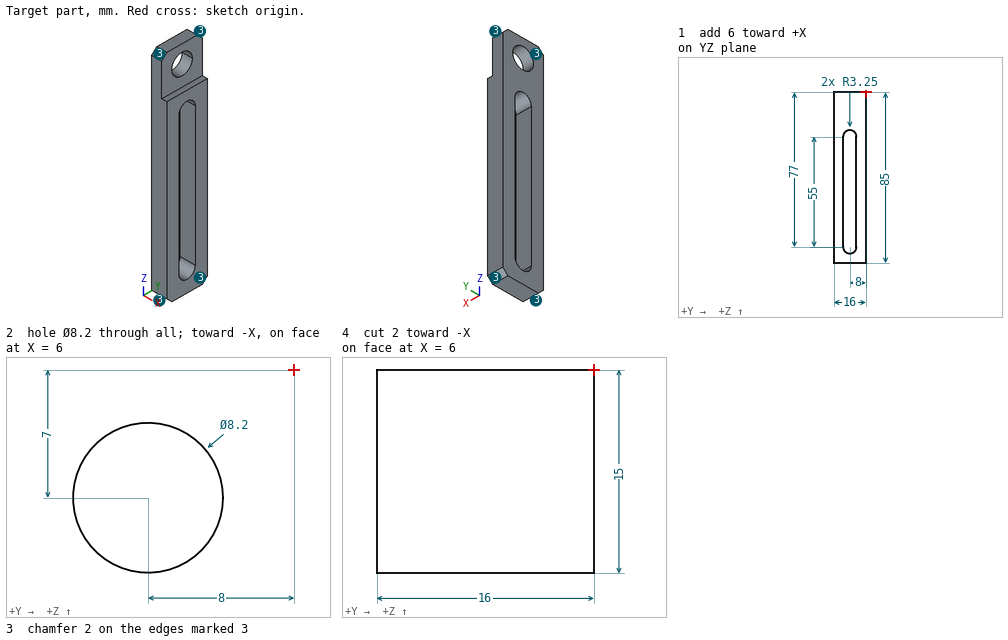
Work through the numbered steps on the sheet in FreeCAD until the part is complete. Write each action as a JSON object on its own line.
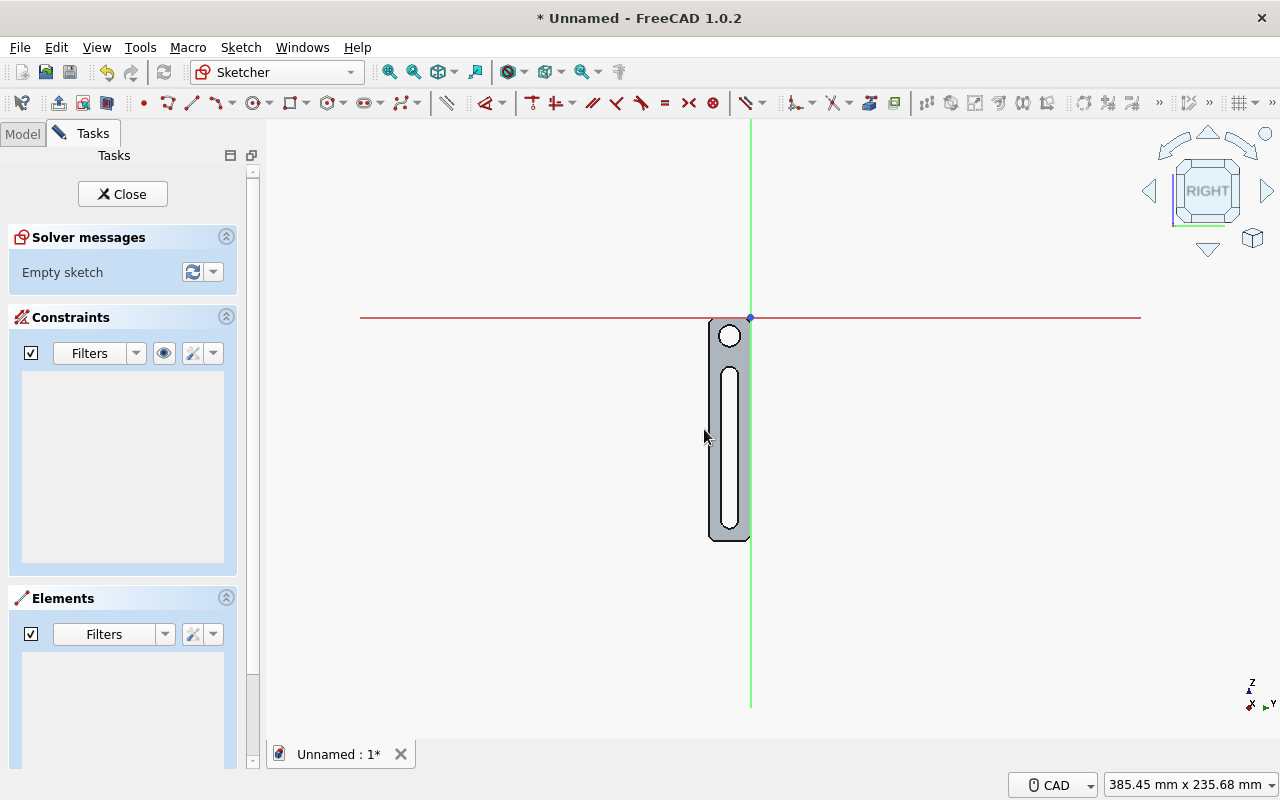
{"action": "scroll", "coordinate": [732, 328], "scroll_direction": "up", "scroll_amount": 12}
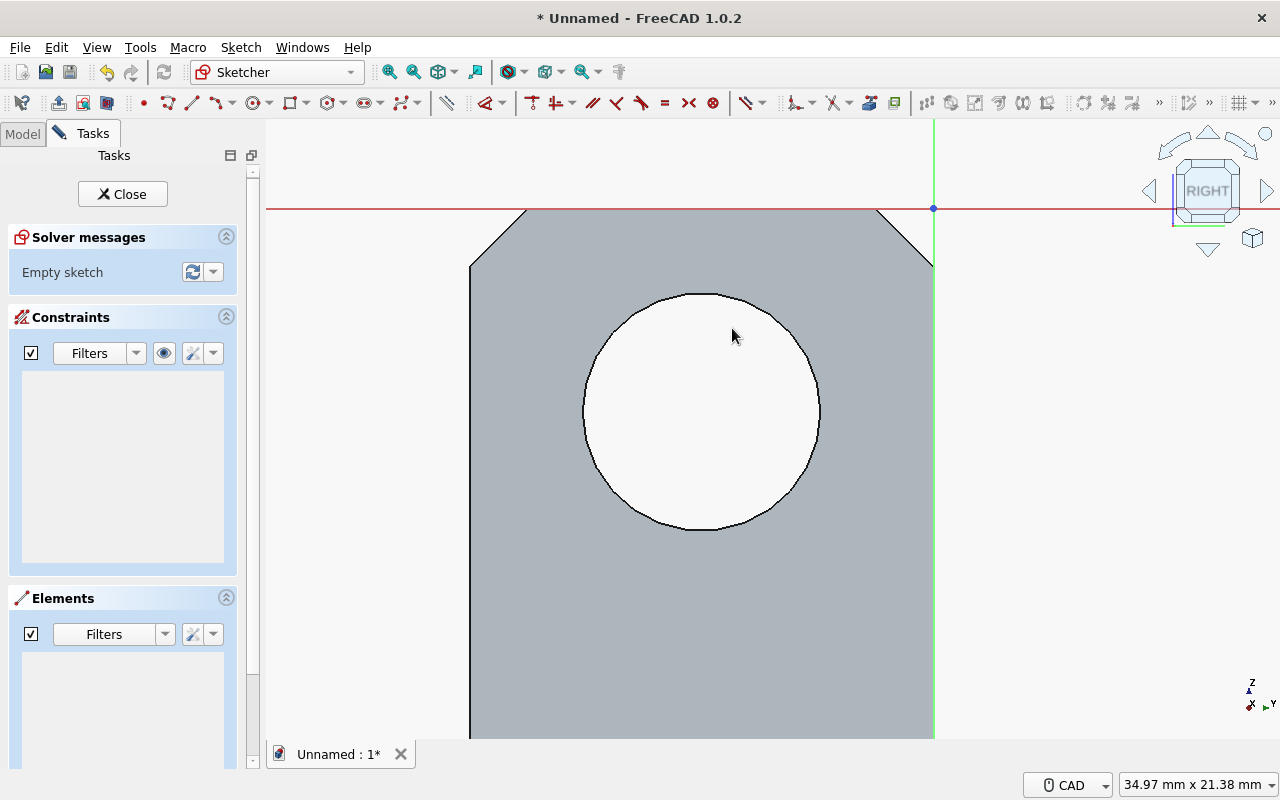
{"action": "key", "text": "g r"}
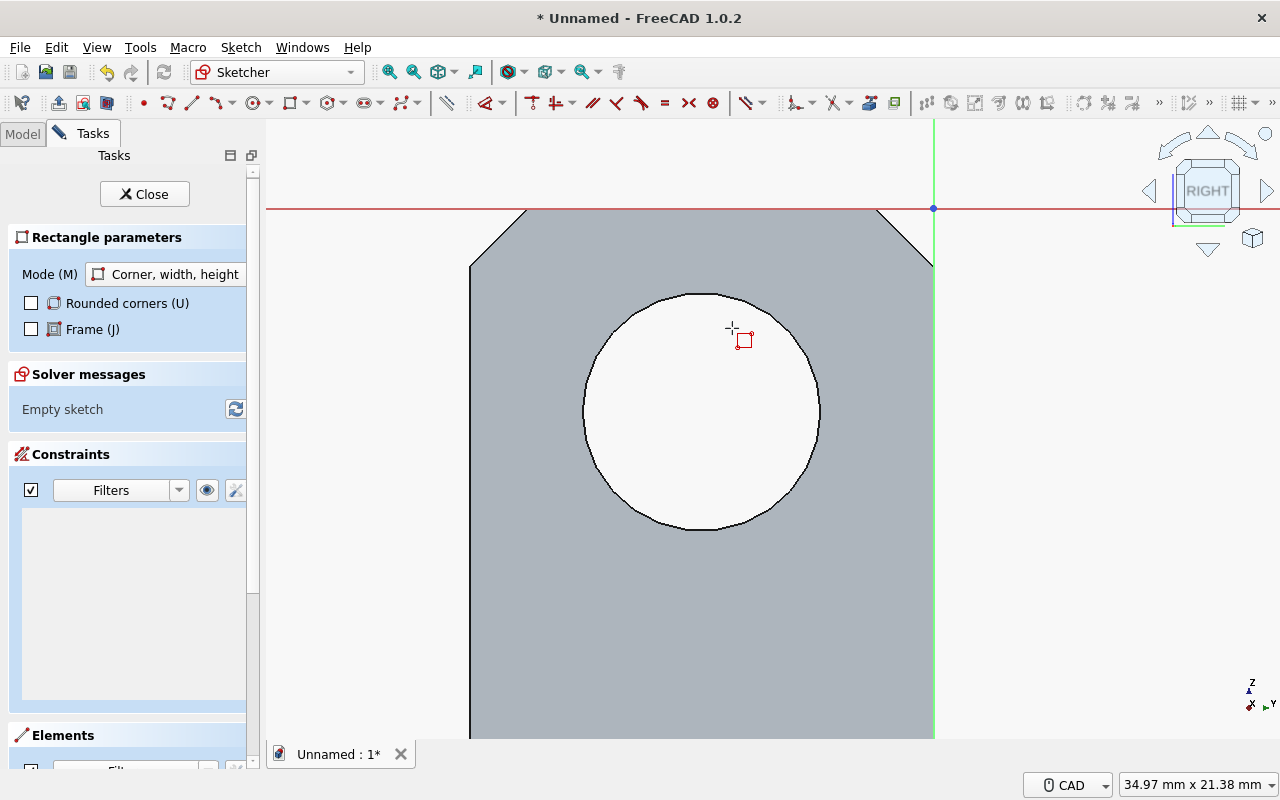
{"action": "left_click", "coordinate": [934, 209]}
{"action": "mouse_move", "coordinate": [470, 644]}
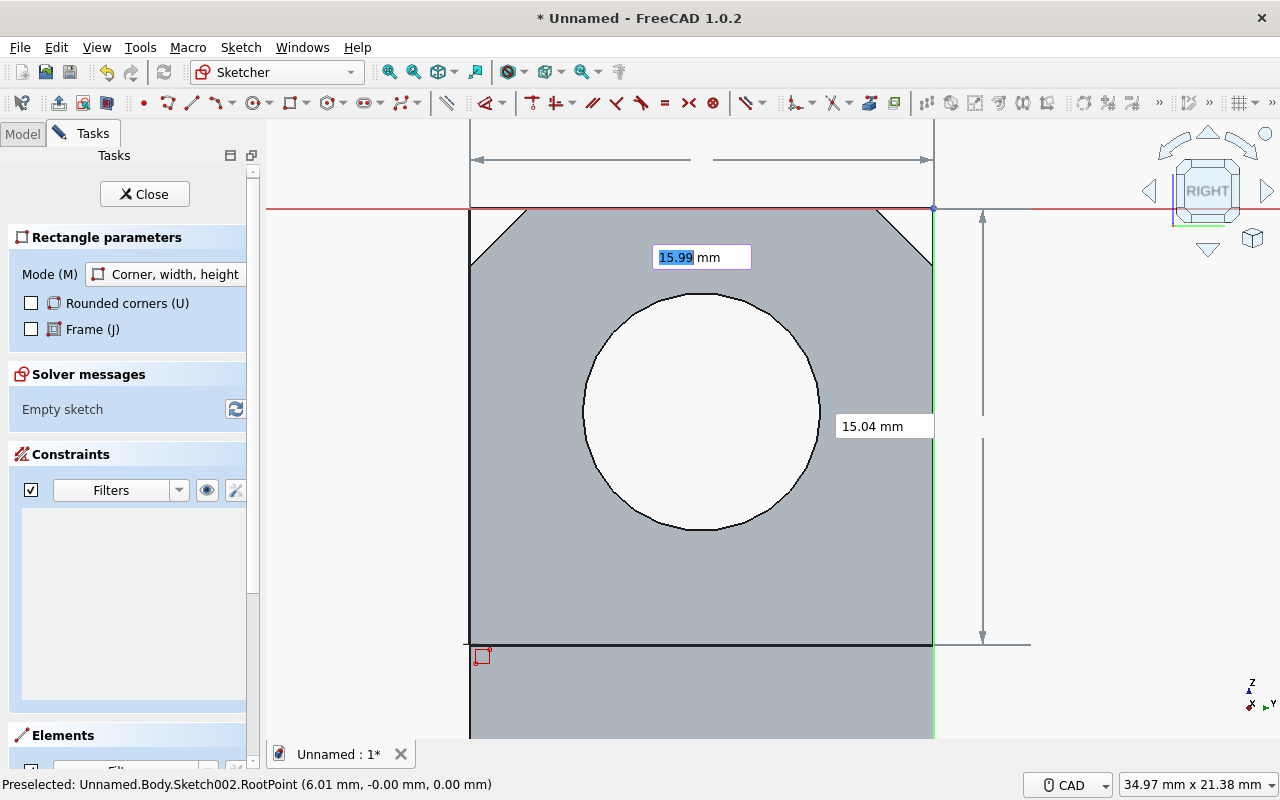
{"action": "type", "text": "16"}
{"action": "key", "text": "Tab"}
{"action": "type", "text": "15"}
{"action": "key", "text": "Return"}
{"action": "key", "text": "Escape"}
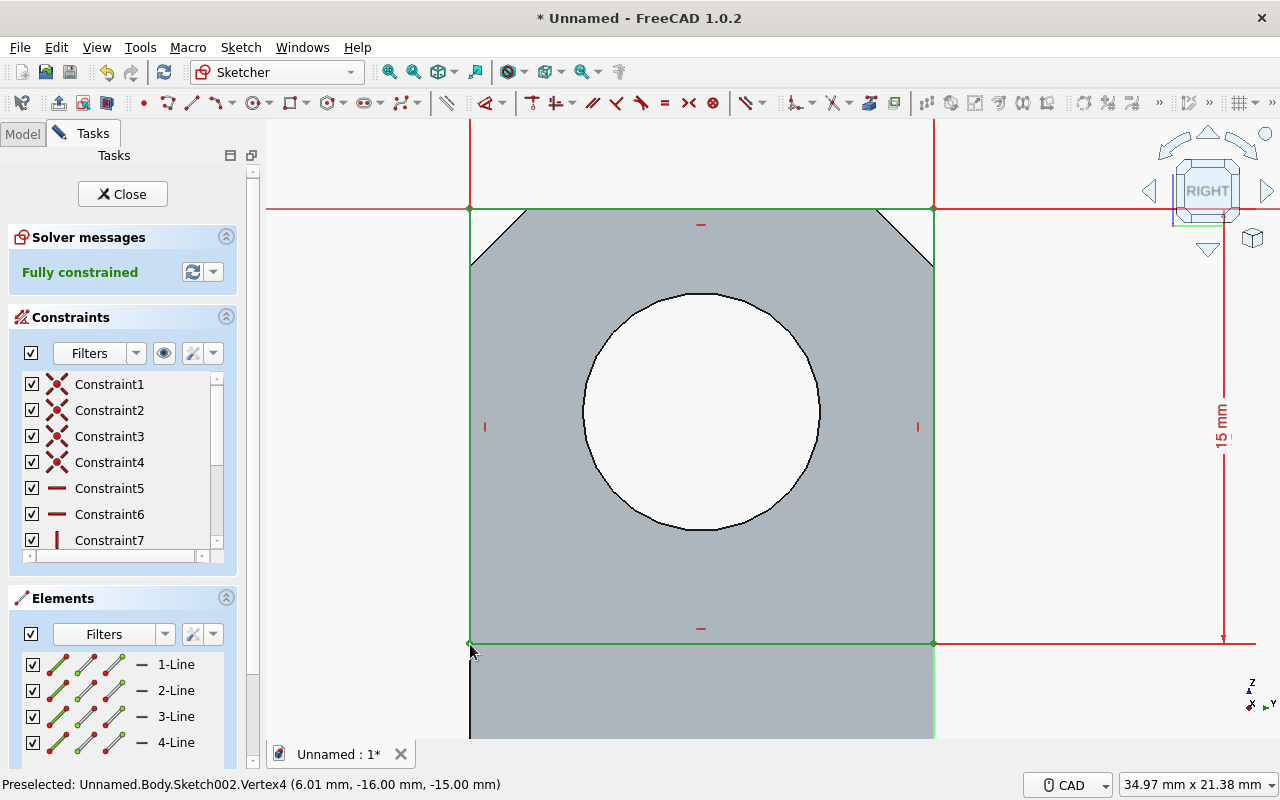
{"action": "left_click", "coordinate": [123, 194]}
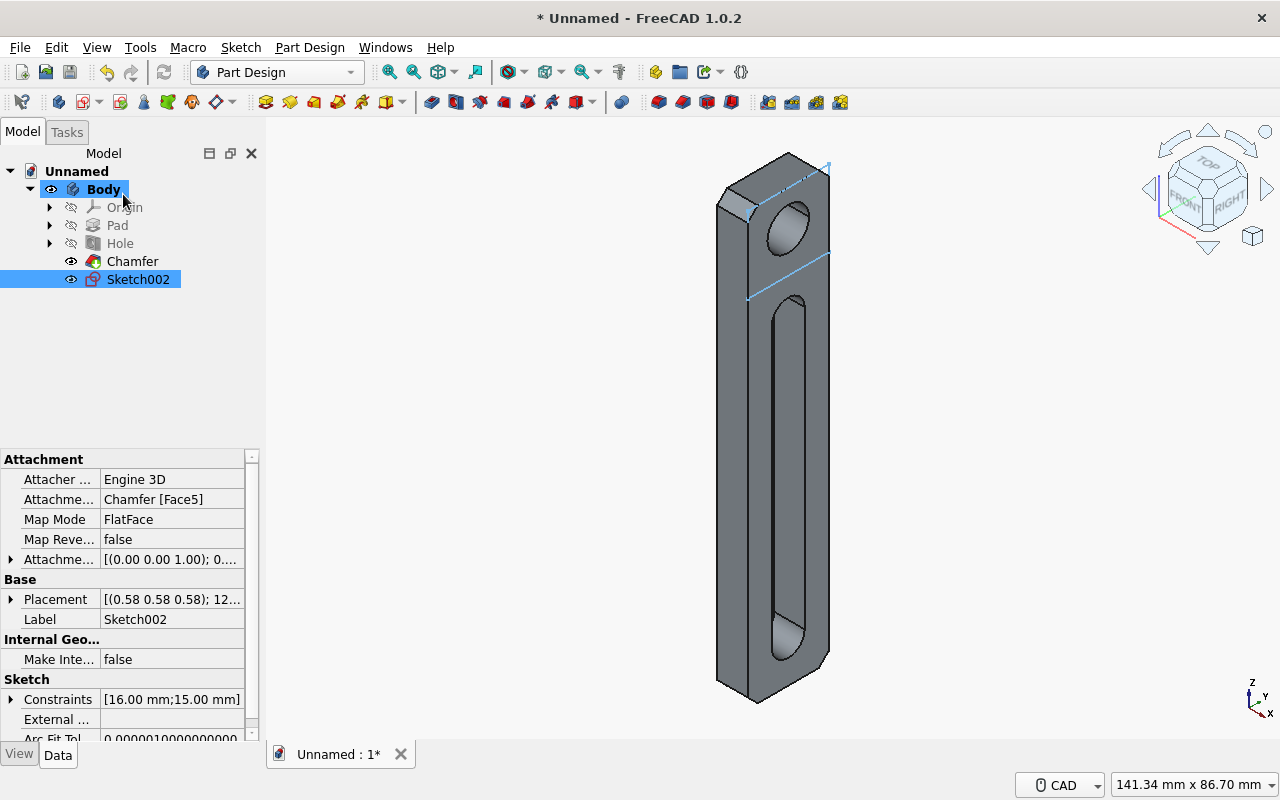
{"action": "left_click", "coordinate": [432, 102]}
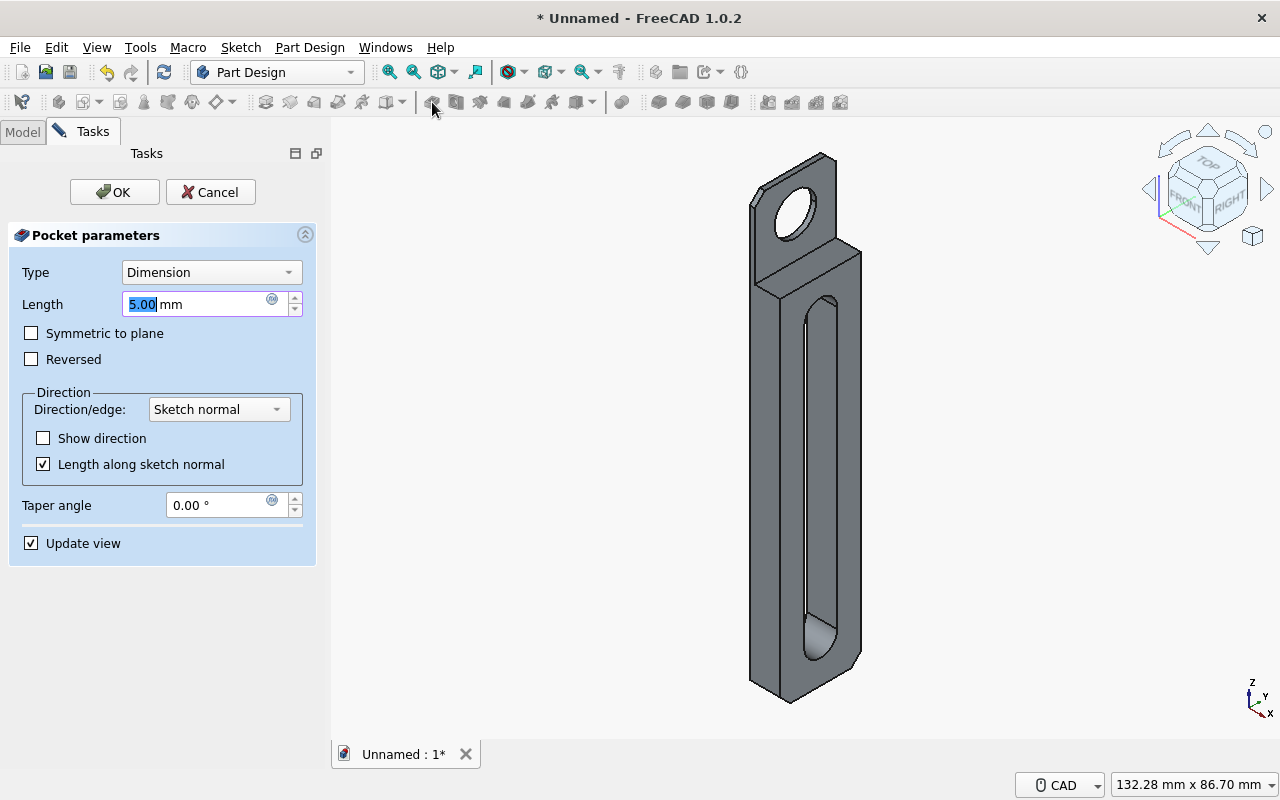
{"action": "type", "text": "2"}
{"action": "key", "text": "Tab"}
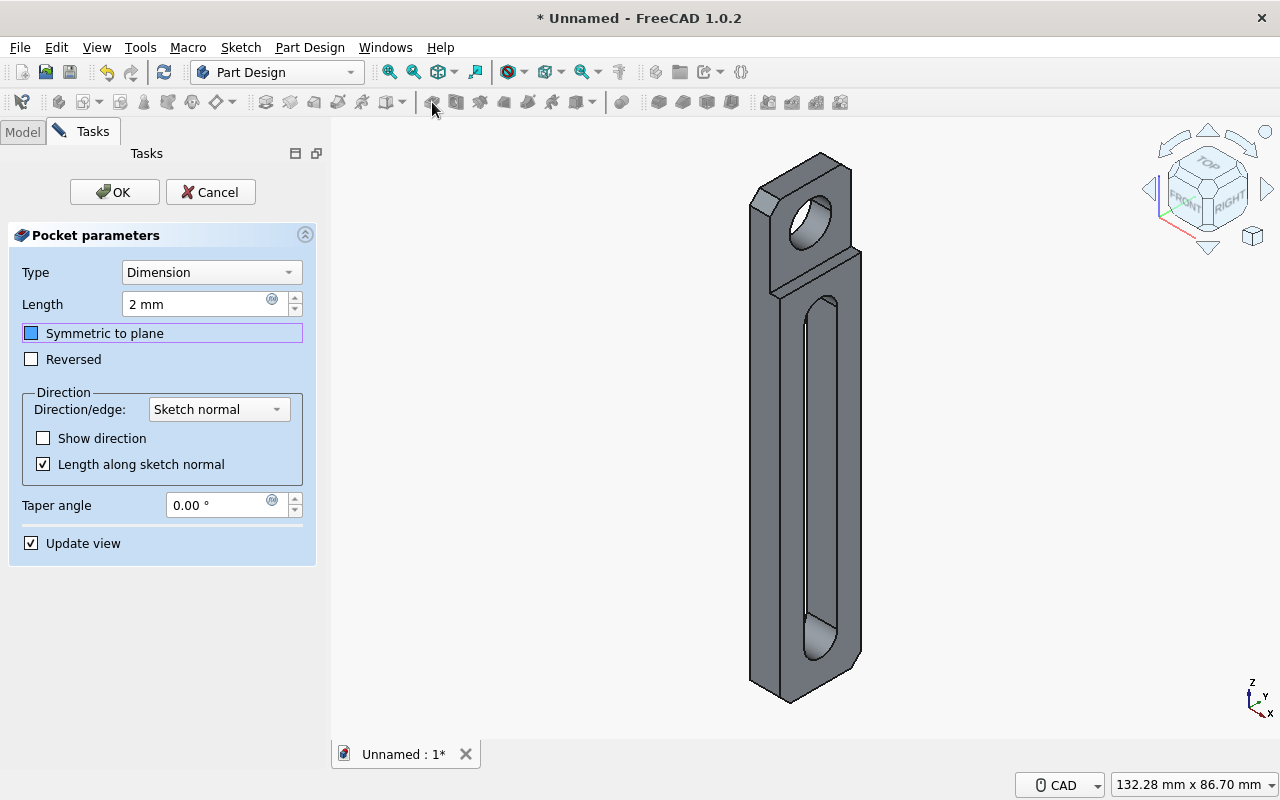
{"action": "left_click", "coordinate": [115, 192]}